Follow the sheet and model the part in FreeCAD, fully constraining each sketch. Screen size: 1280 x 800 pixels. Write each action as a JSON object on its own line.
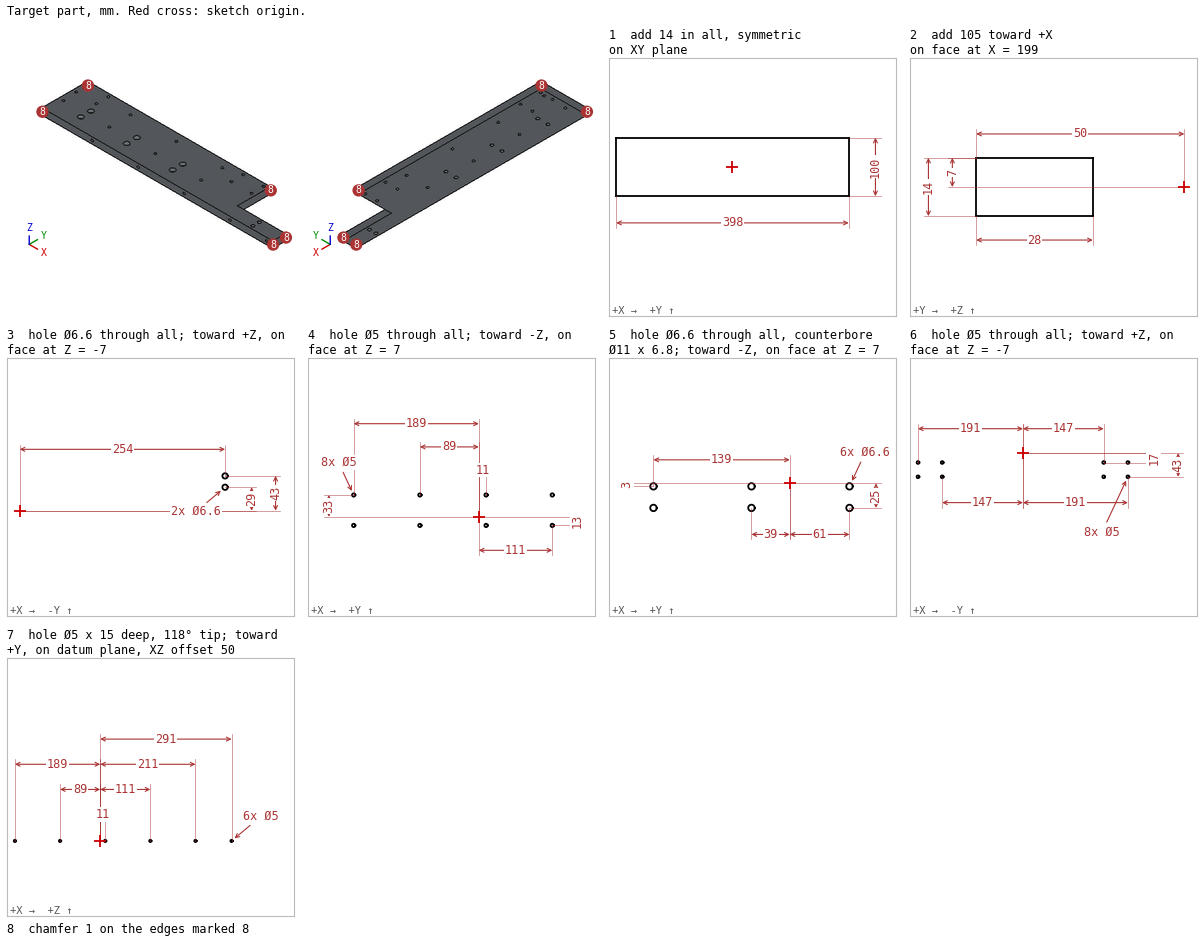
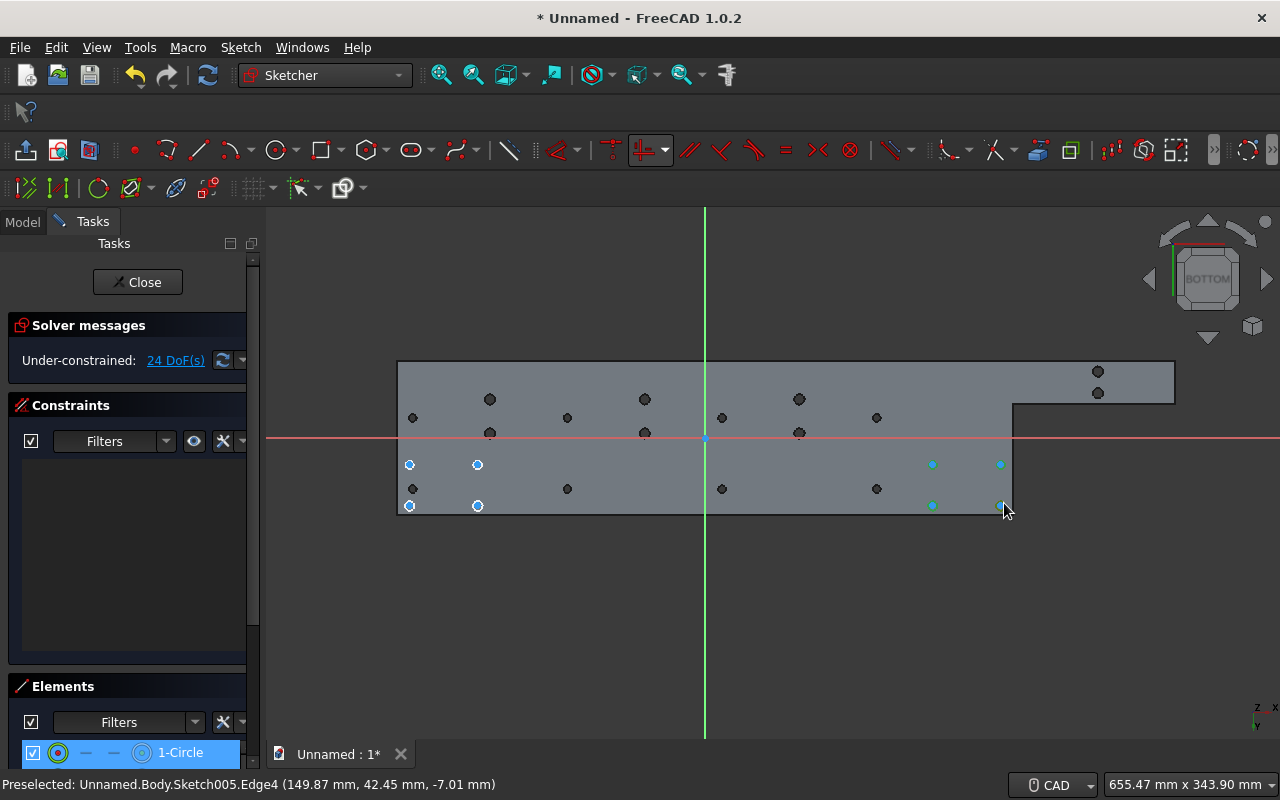
{"action": "scroll", "coordinate": [481, 503], "scroll_direction": "up", "scroll_amount": 6}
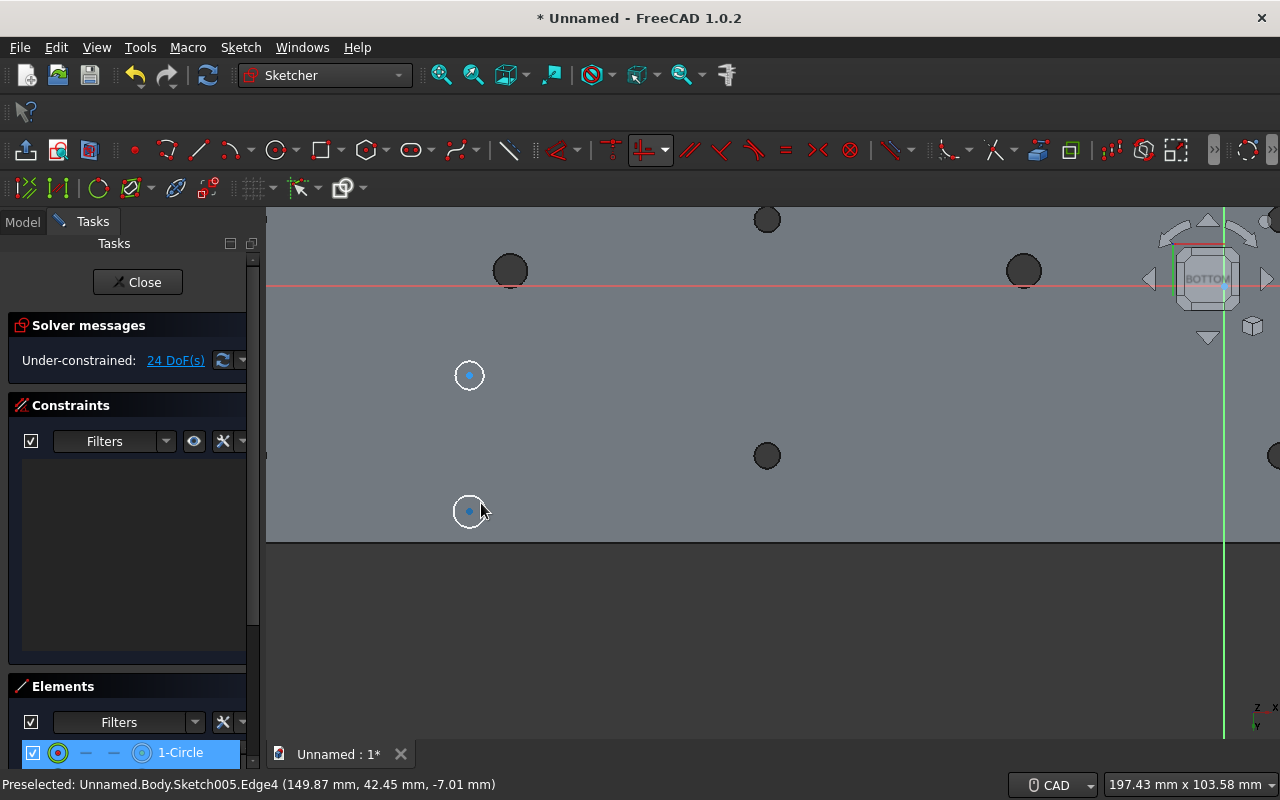
{"action": "left_click", "coordinate": [481, 500]}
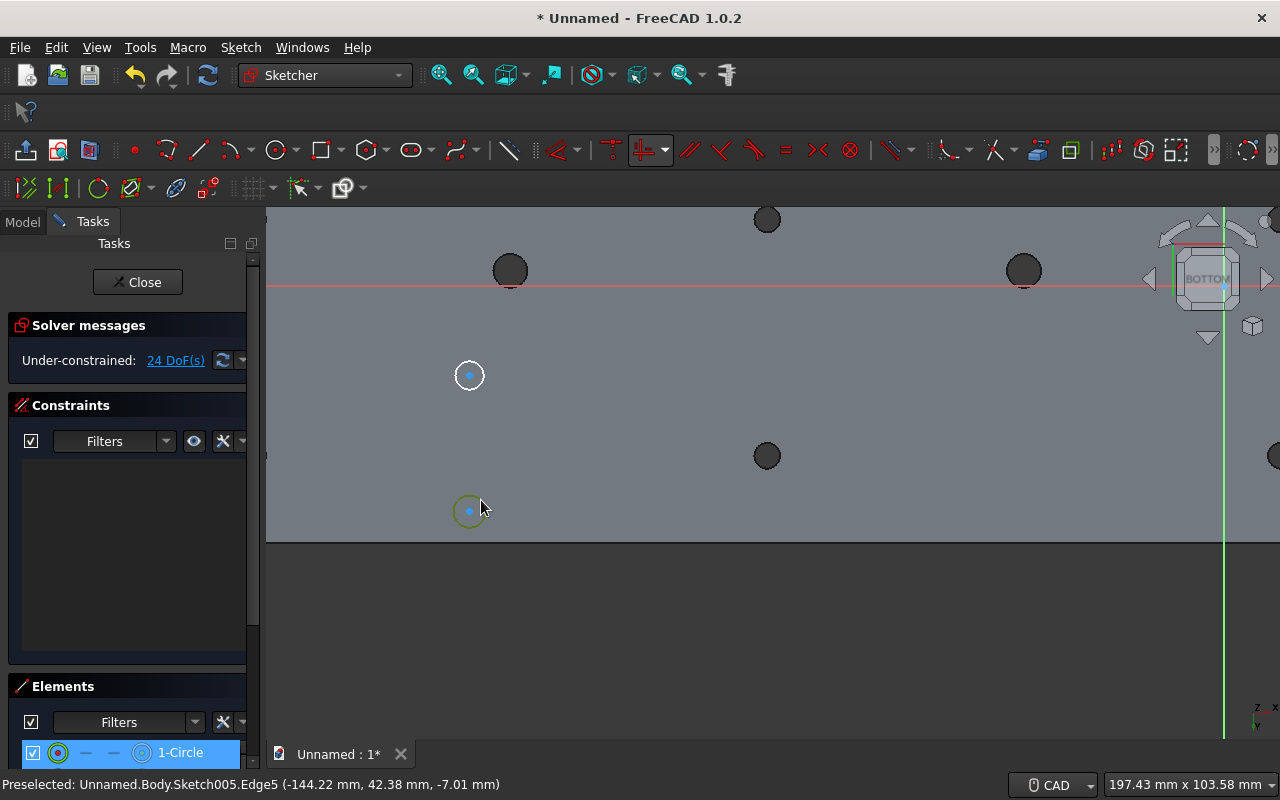
{"action": "scroll", "coordinate": [480, 503], "scroll_direction": "down", "scroll_amount": 6}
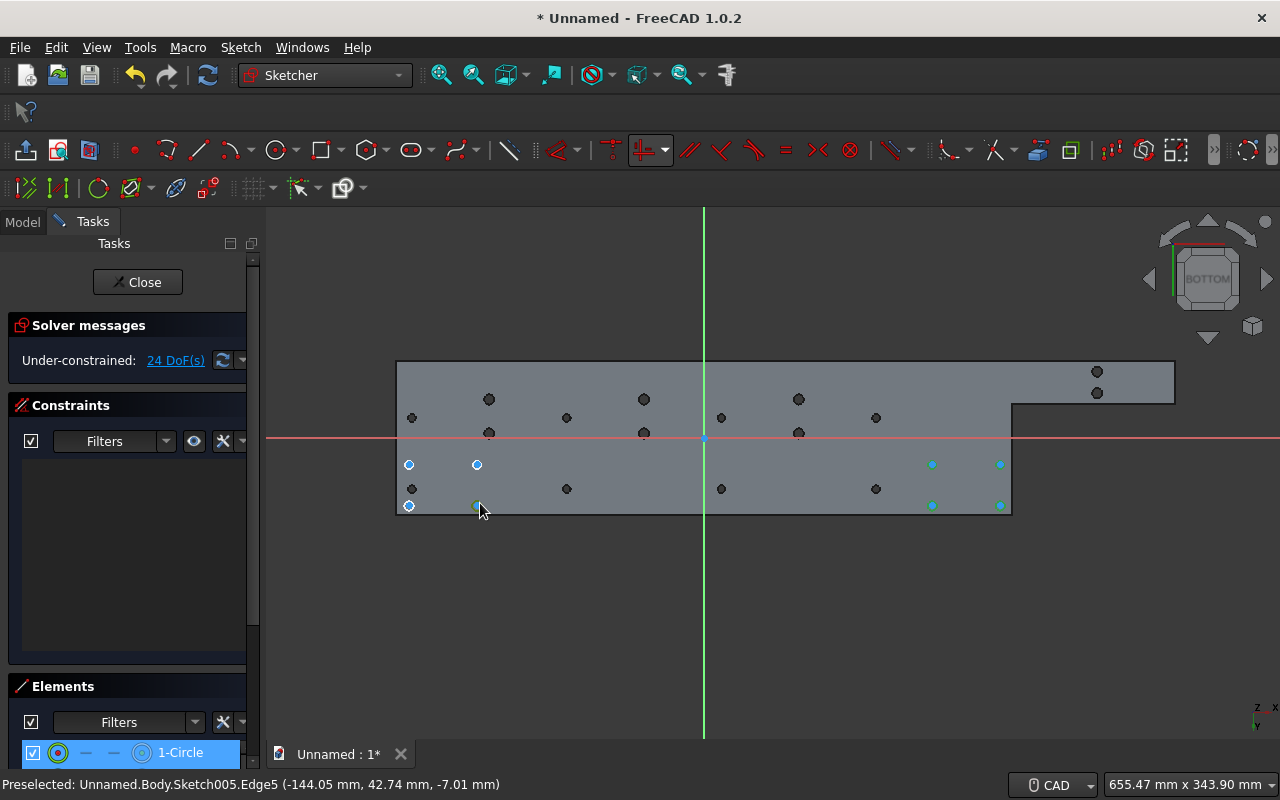
{"action": "scroll", "coordinate": [412, 462], "scroll_direction": "up", "scroll_amount": 7}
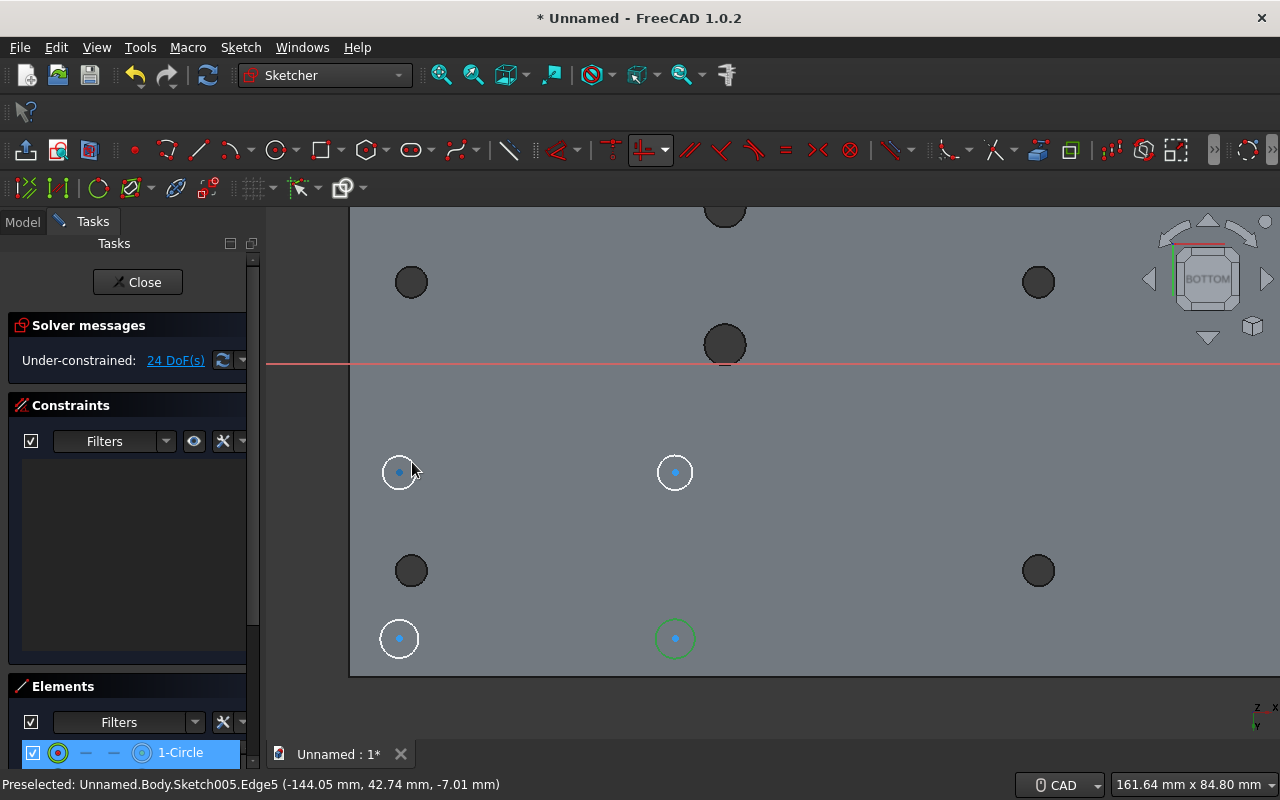
{"action": "left_click", "coordinate": [411, 461]}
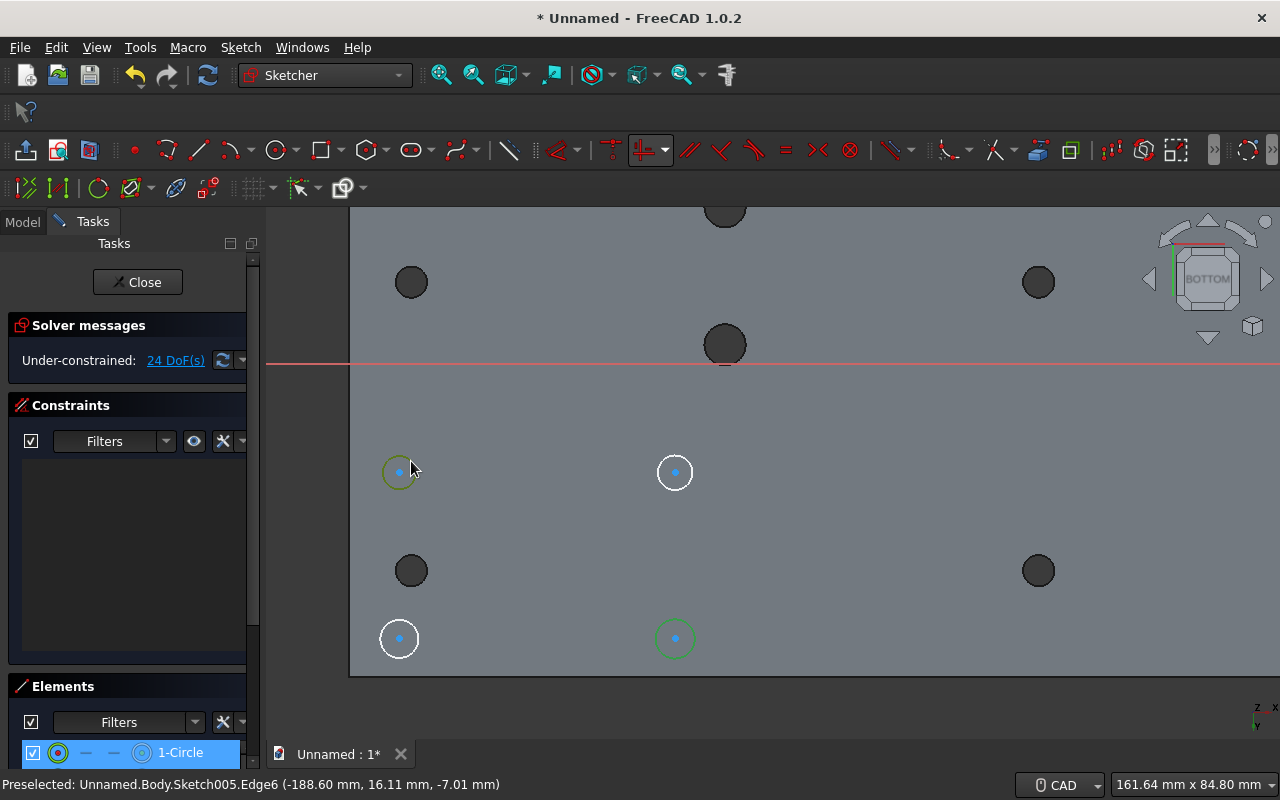
{"action": "left_click", "coordinate": [687, 460]}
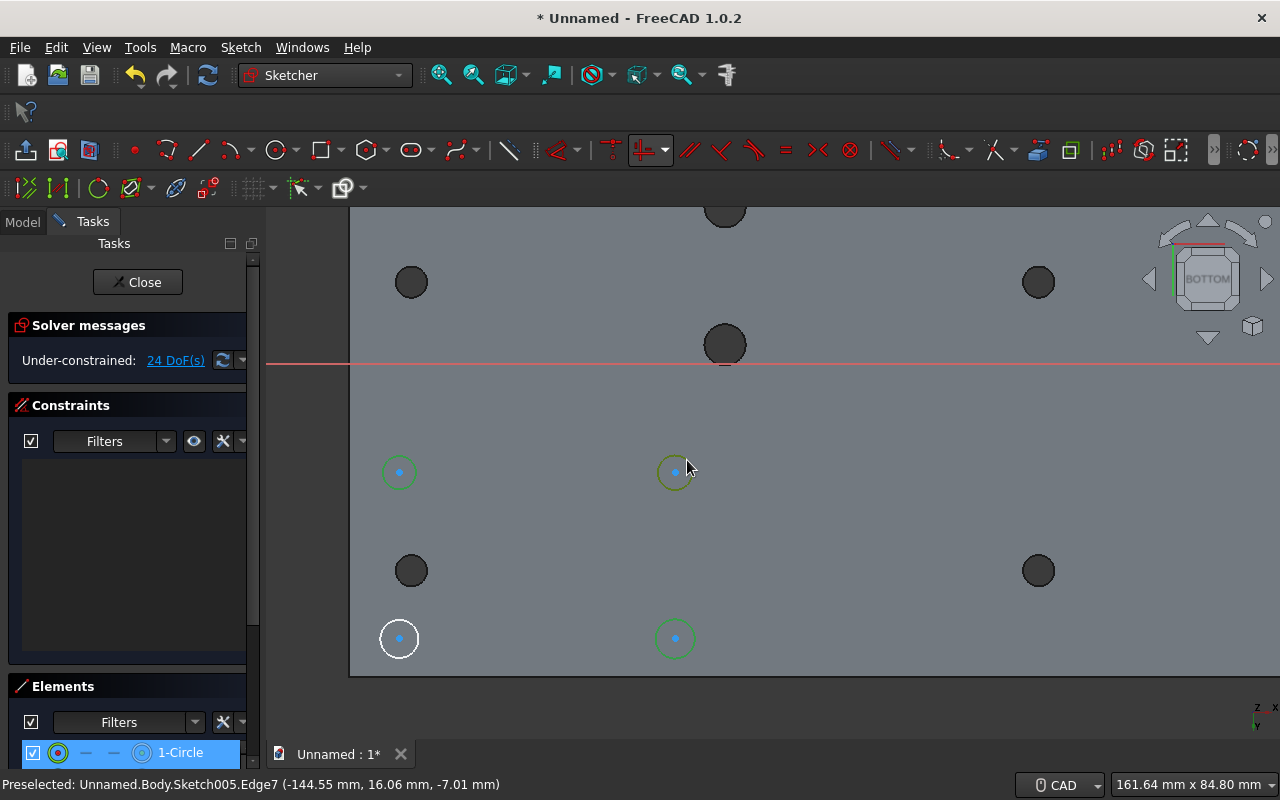
{"action": "left_click", "coordinate": [413, 625]}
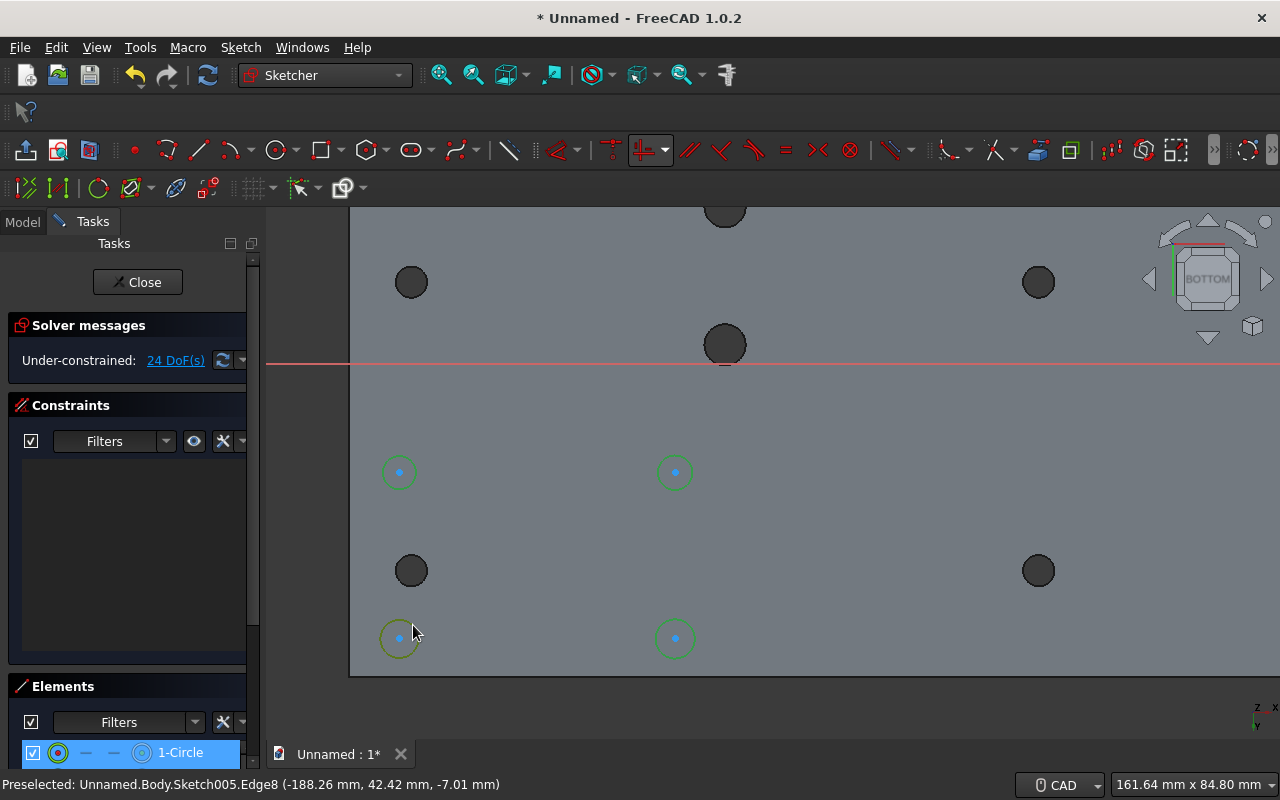
{"action": "left_click", "coordinate": [786, 150]}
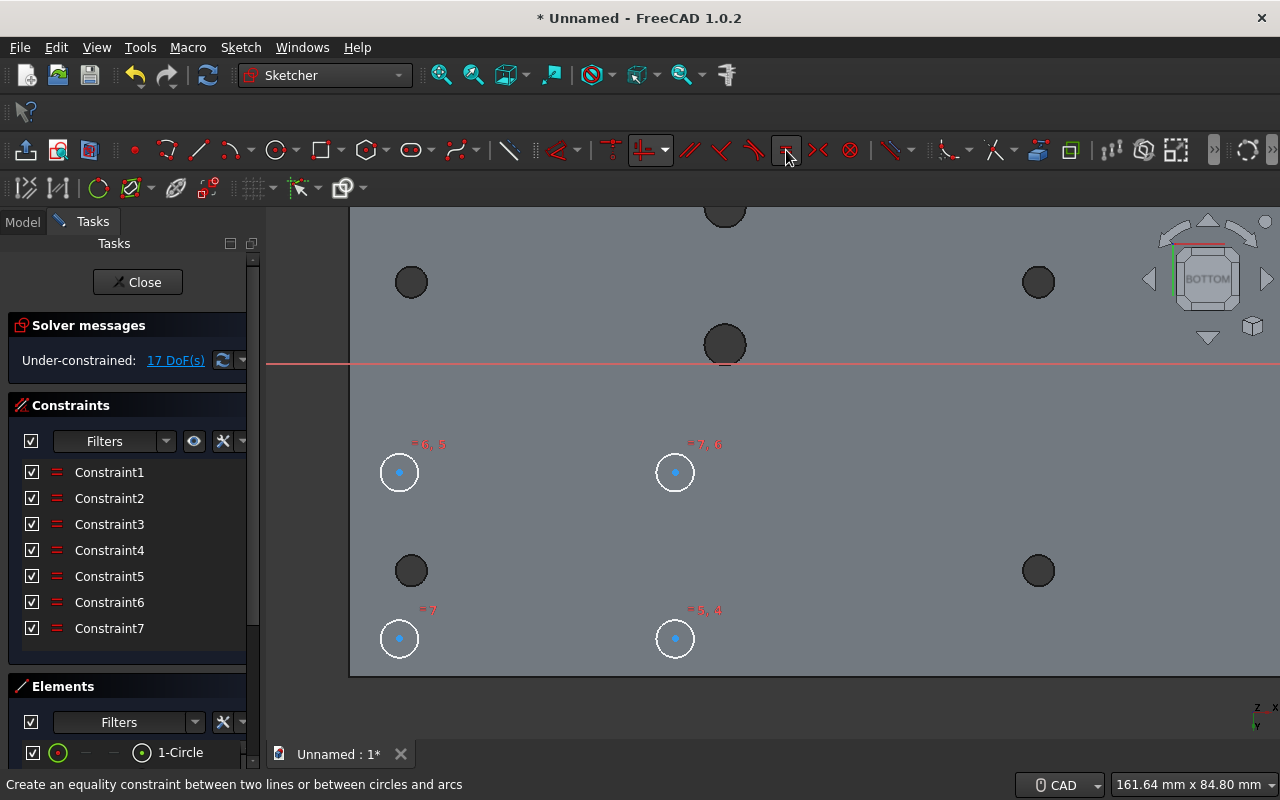
{"action": "scroll", "coordinate": [412, 462], "scroll_direction": "down", "scroll_amount": 7}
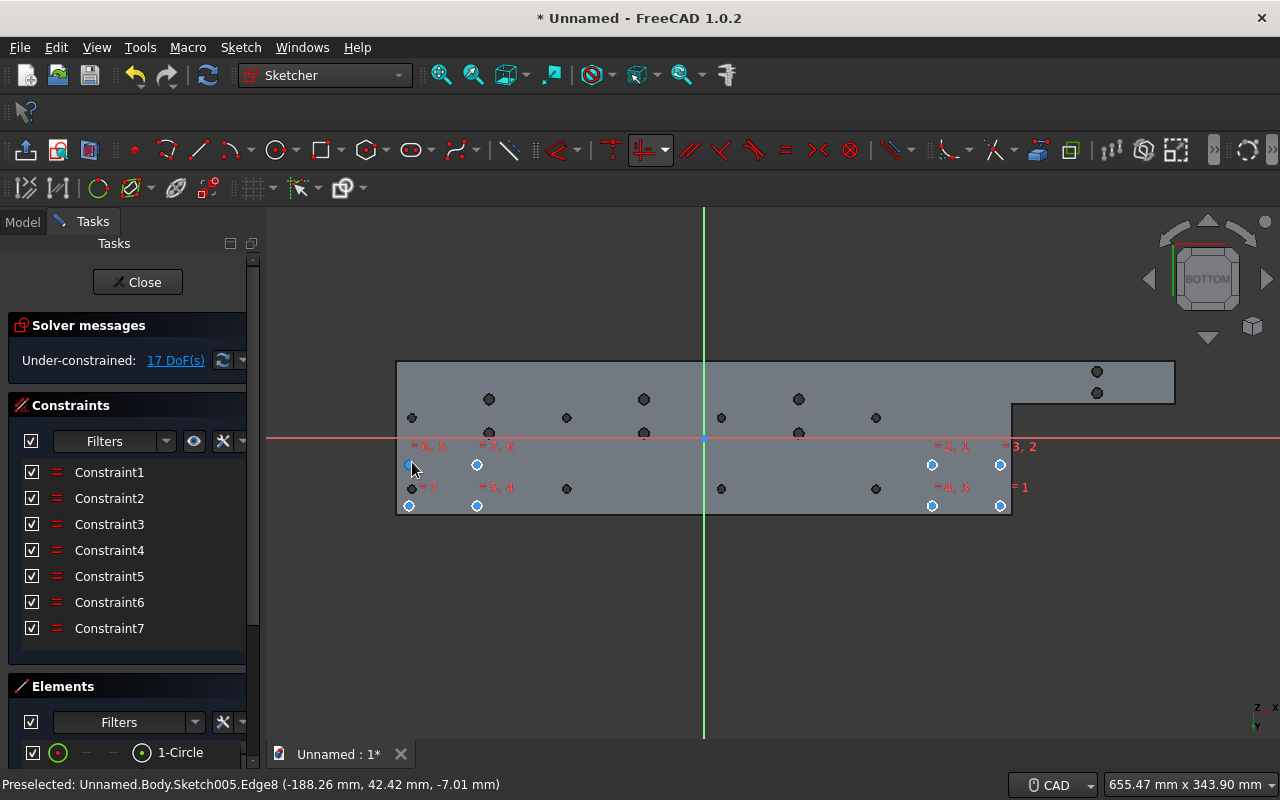
{"action": "left_click", "coordinate": [1000, 506]}